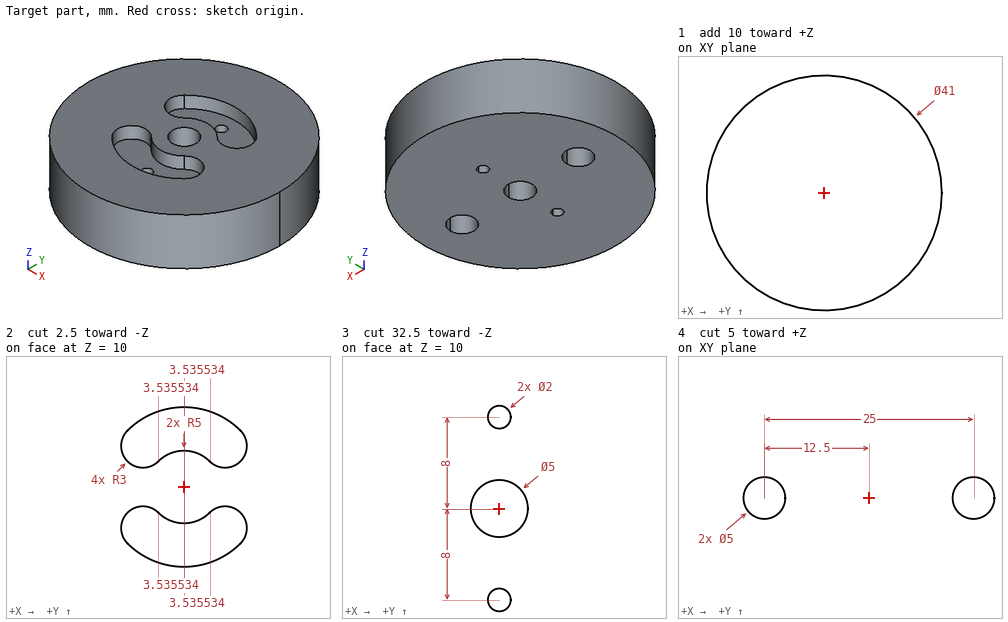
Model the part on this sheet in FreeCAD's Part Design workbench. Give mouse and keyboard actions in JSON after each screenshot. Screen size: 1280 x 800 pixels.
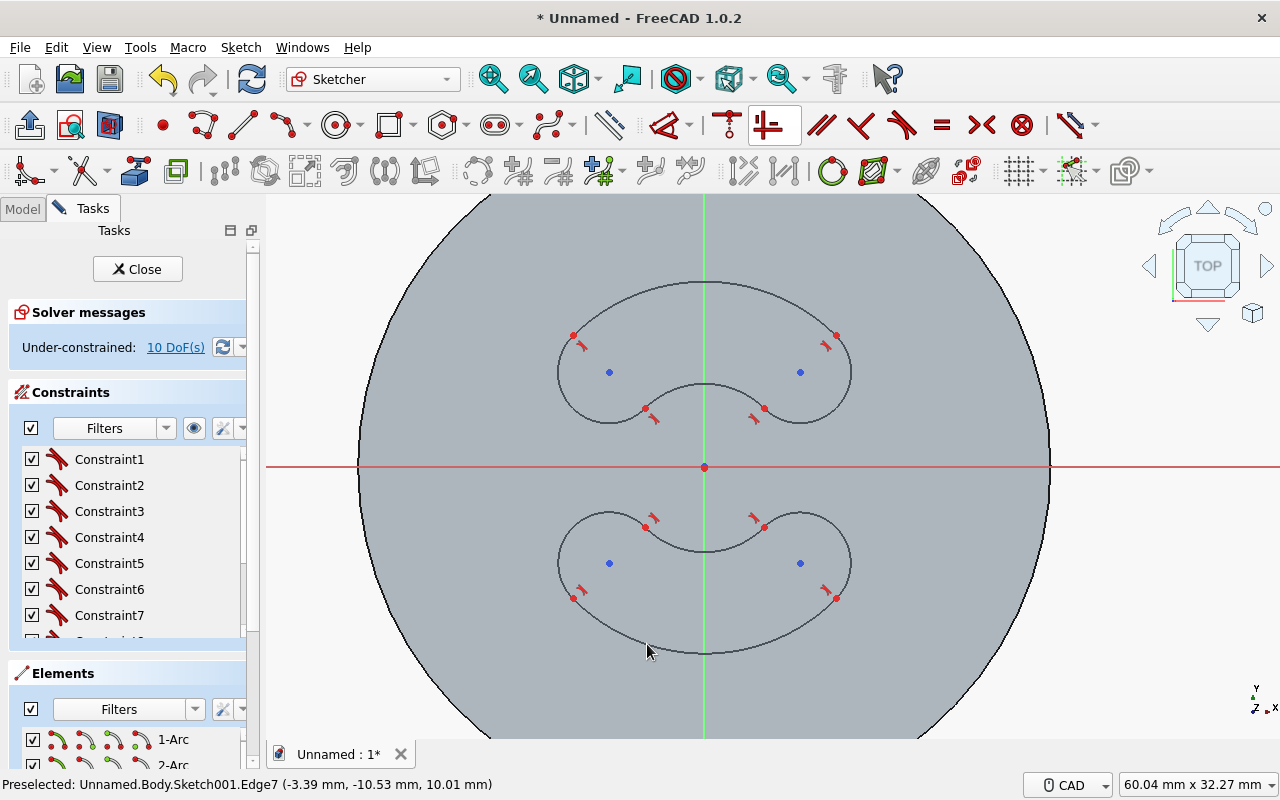
{"action": "left_click_drag", "start_coordinate": [694, 456], "coordinate": [715, 478]}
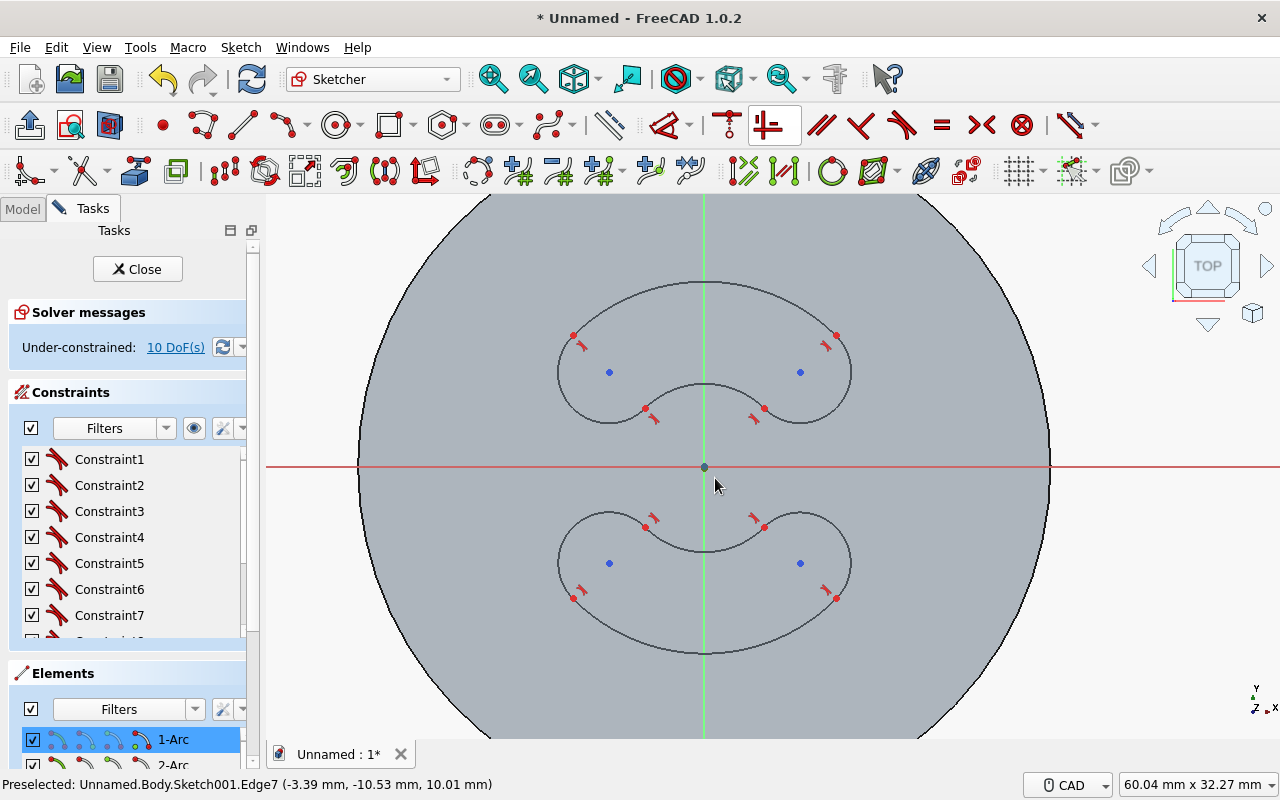
{"action": "key", "text": "c"}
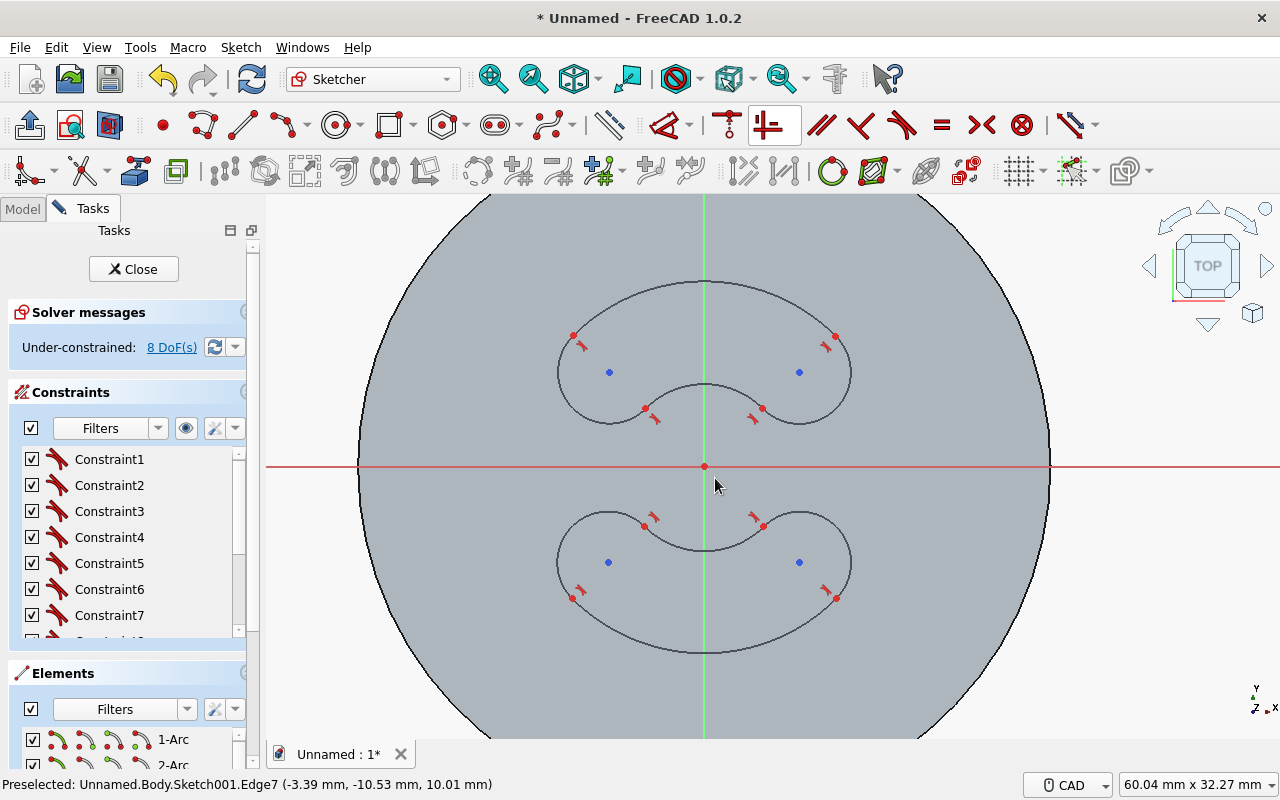
{"action": "left_click", "coordinate": [730, 388]}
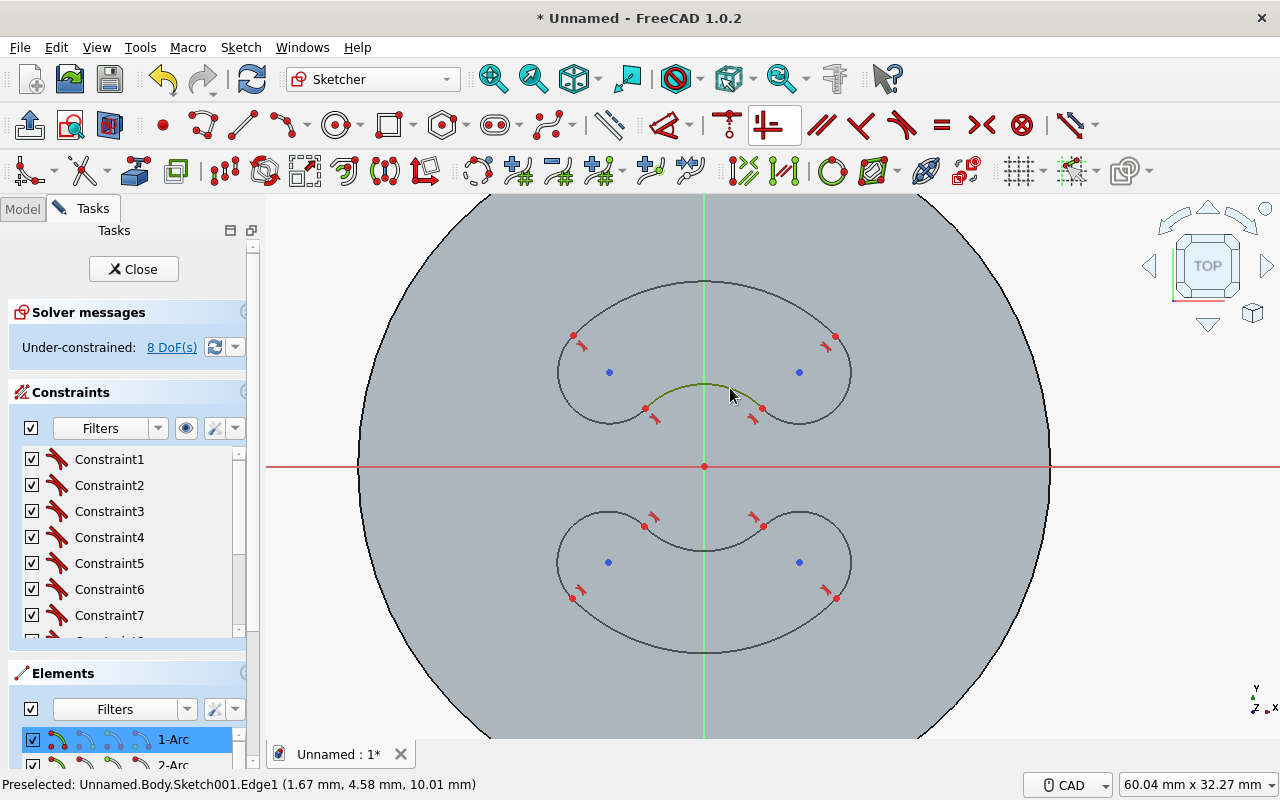
{"action": "left_click", "coordinate": [678, 547]}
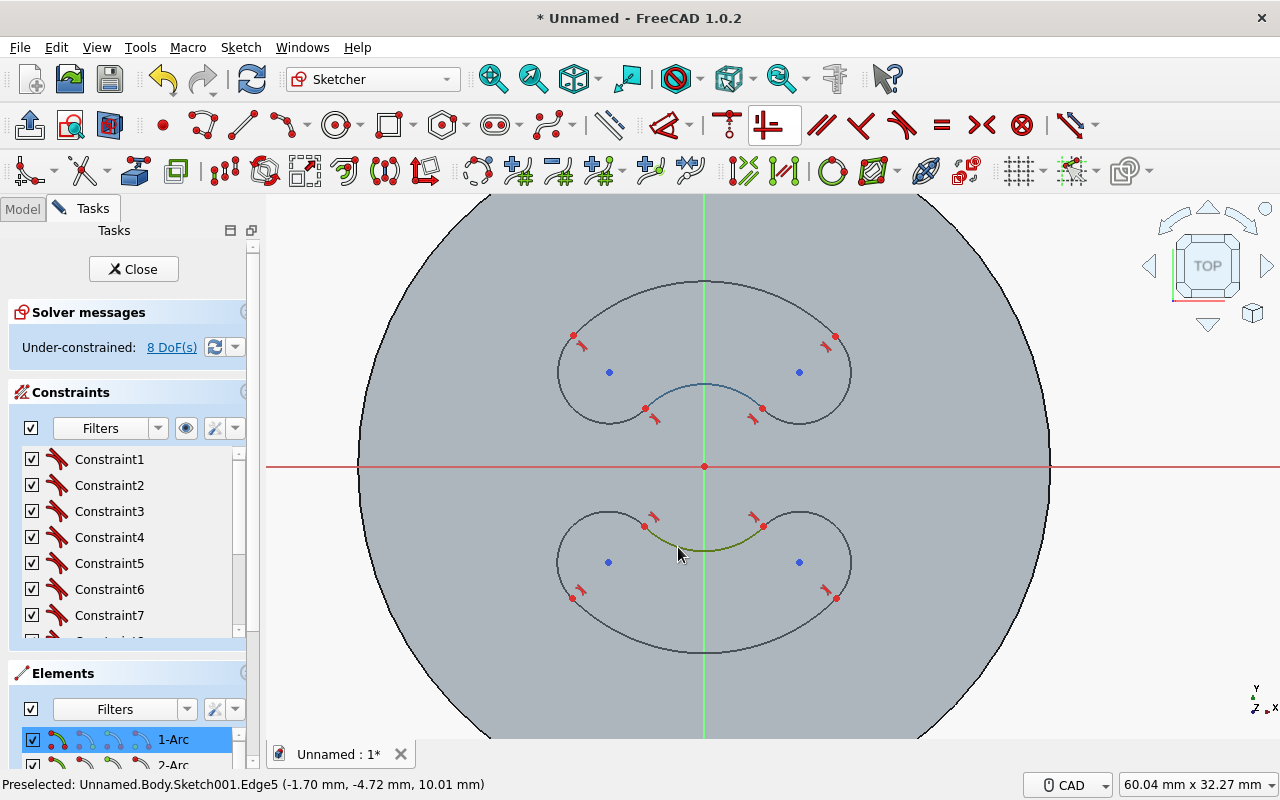
{"action": "key", "text": "e"}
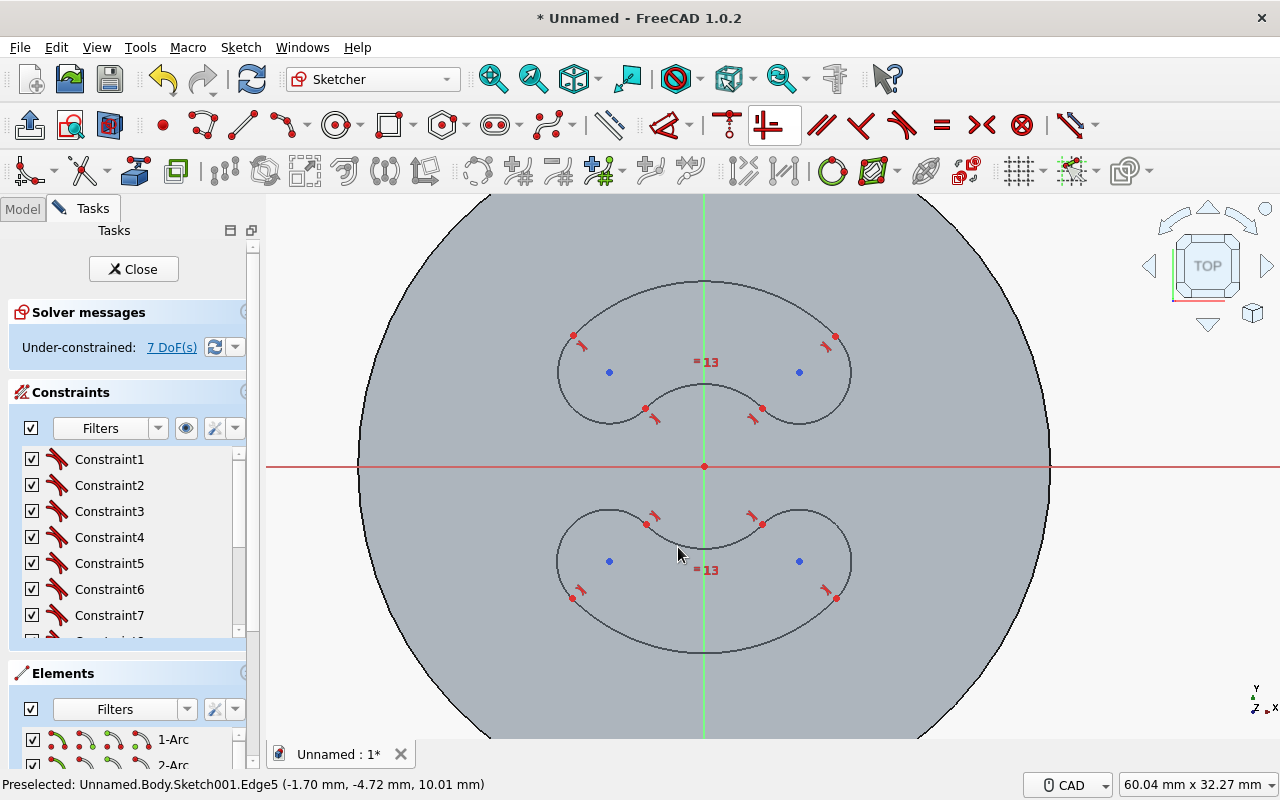
{"action": "left_click", "coordinate": [807, 423]}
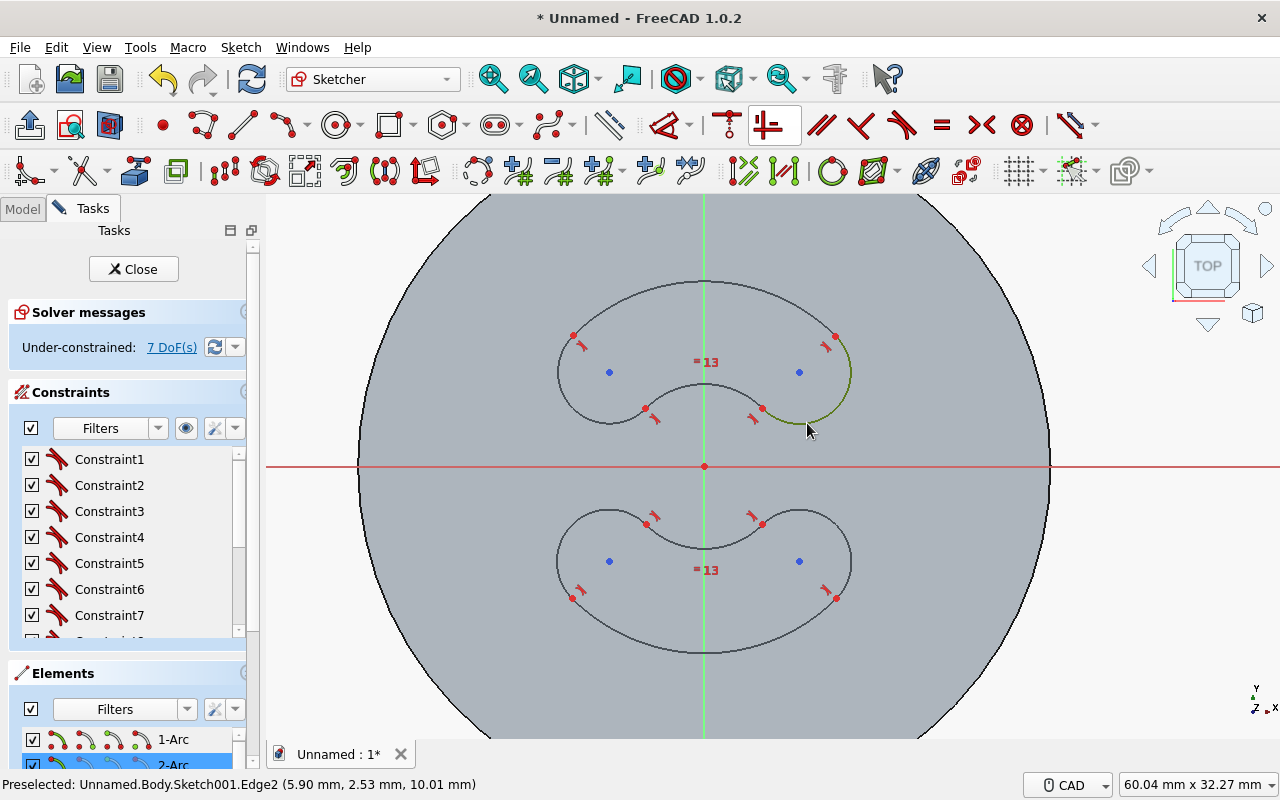
{"action": "left_click", "coordinate": [601, 510]}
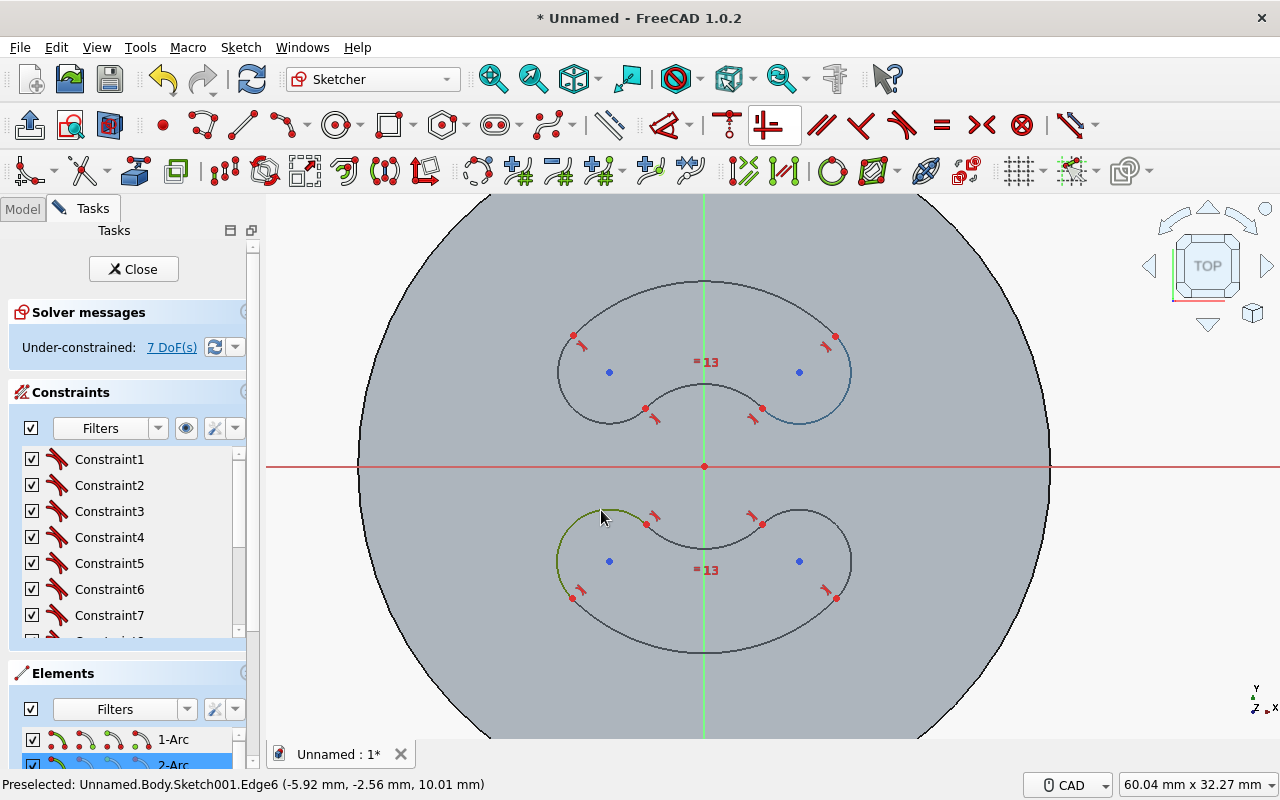
{"action": "left_click", "coordinate": [942, 126]}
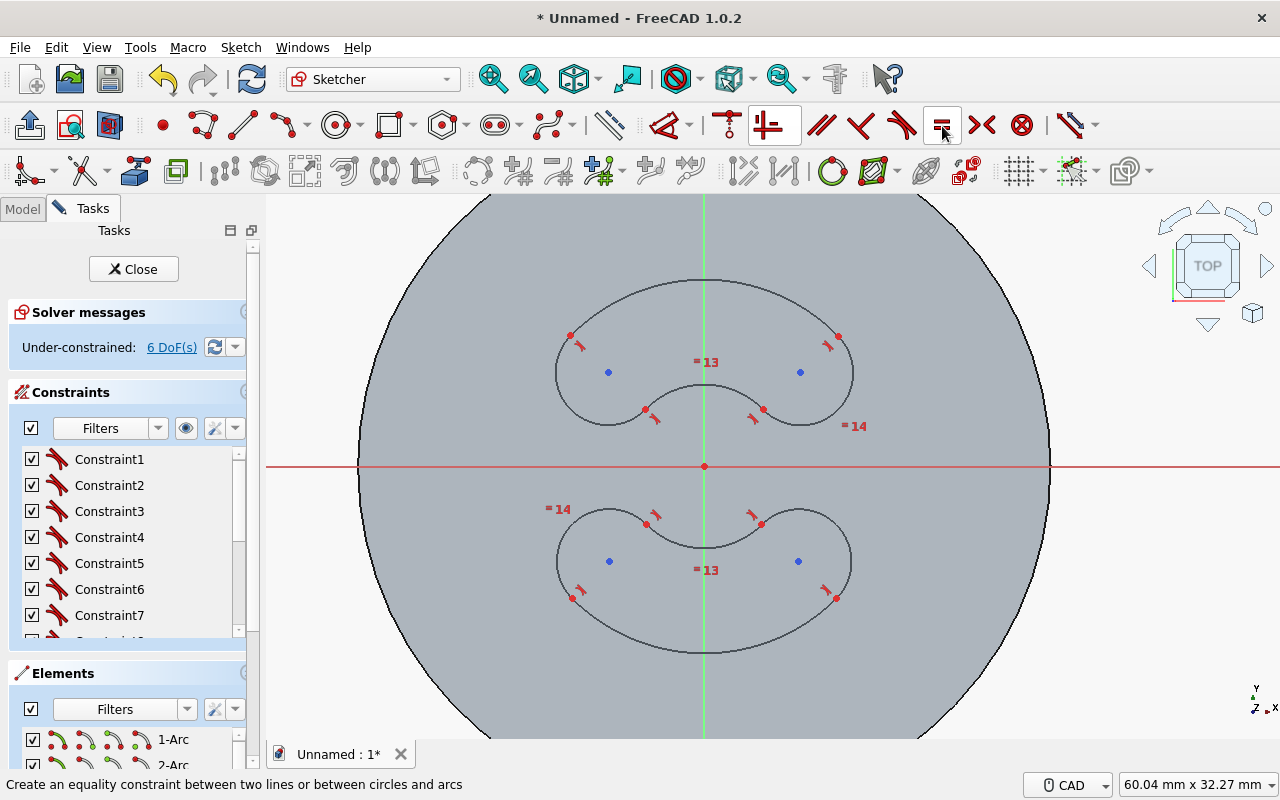
{"action": "left_click", "coordinate": [664, 126]}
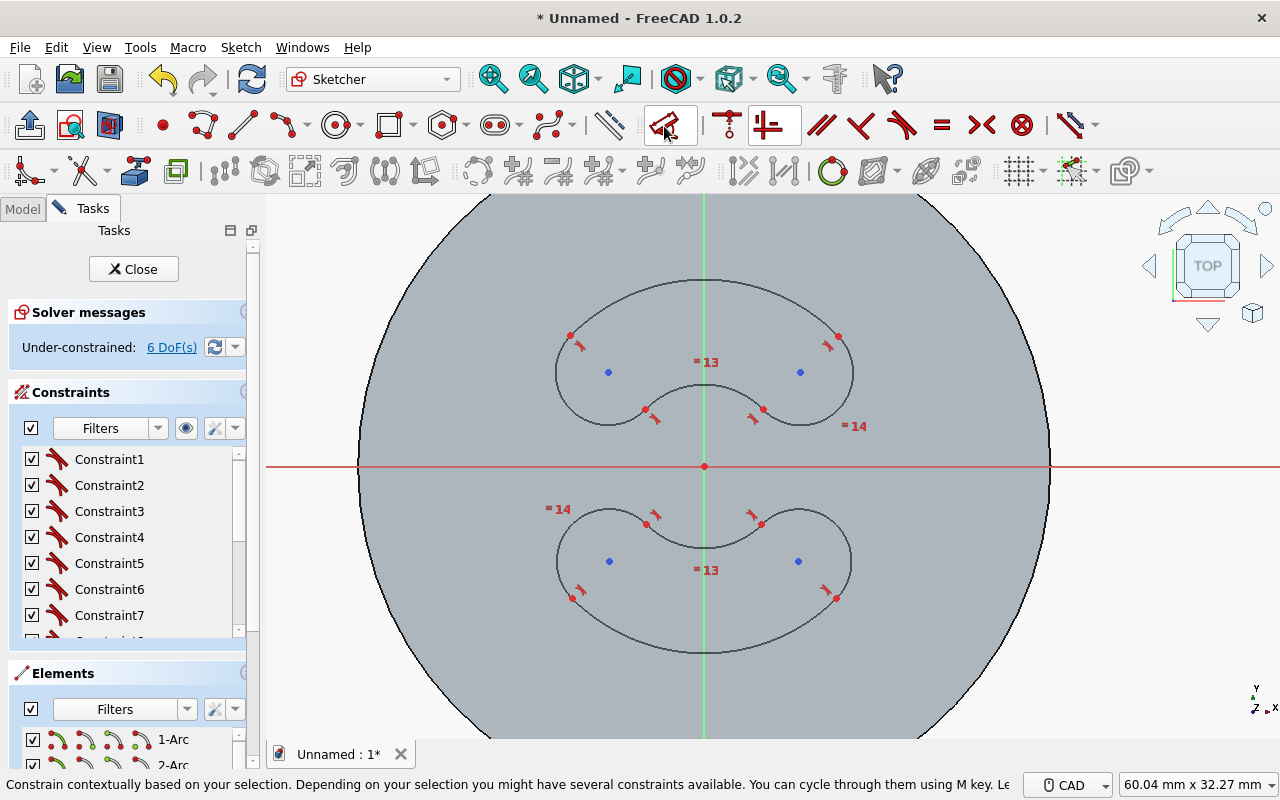
{"action": "left_click", "coordinate": [730, 389]}
{"action": "left_click", "coordinate": [740, 359]}